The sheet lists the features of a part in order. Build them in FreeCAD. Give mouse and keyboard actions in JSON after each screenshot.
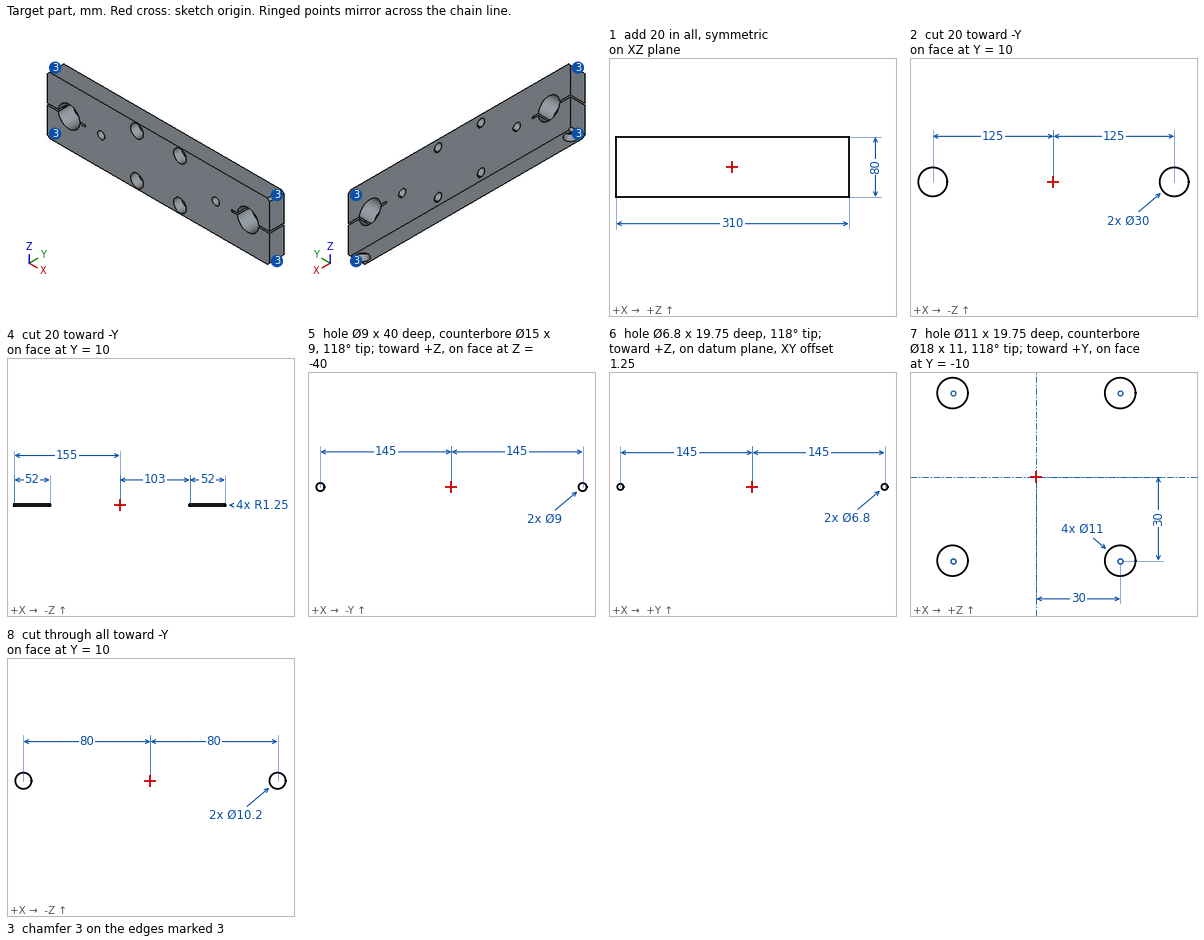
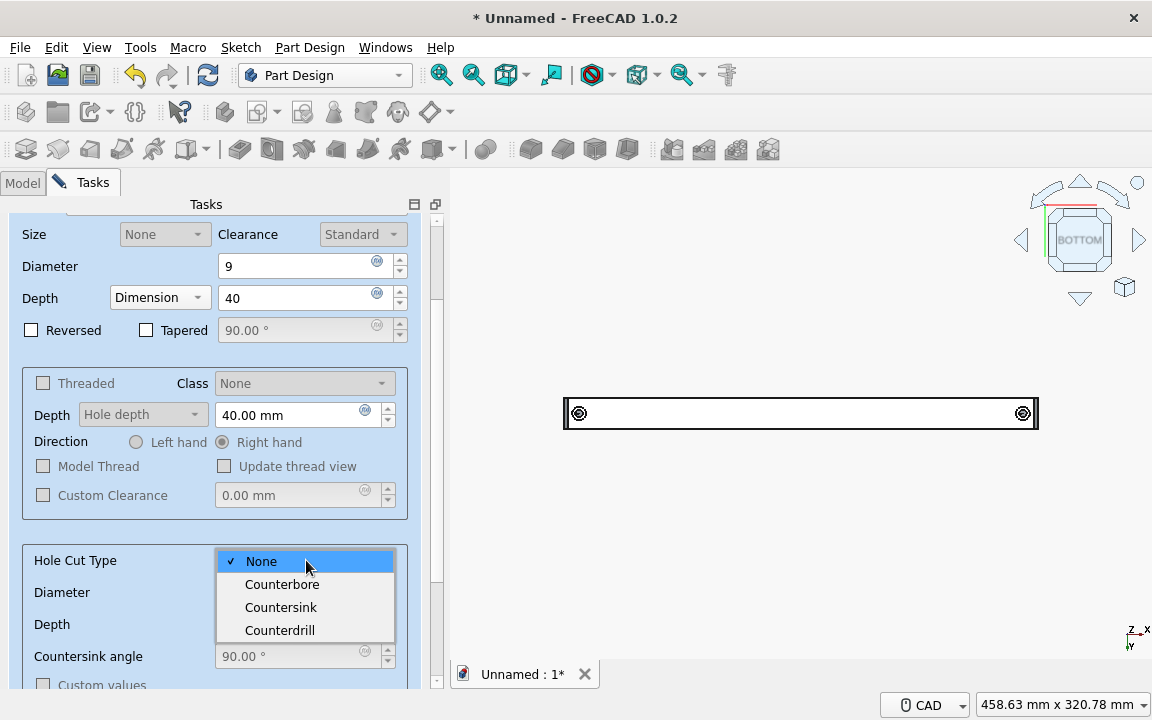
{"action": "left_click", "coordinate": [304, 584]}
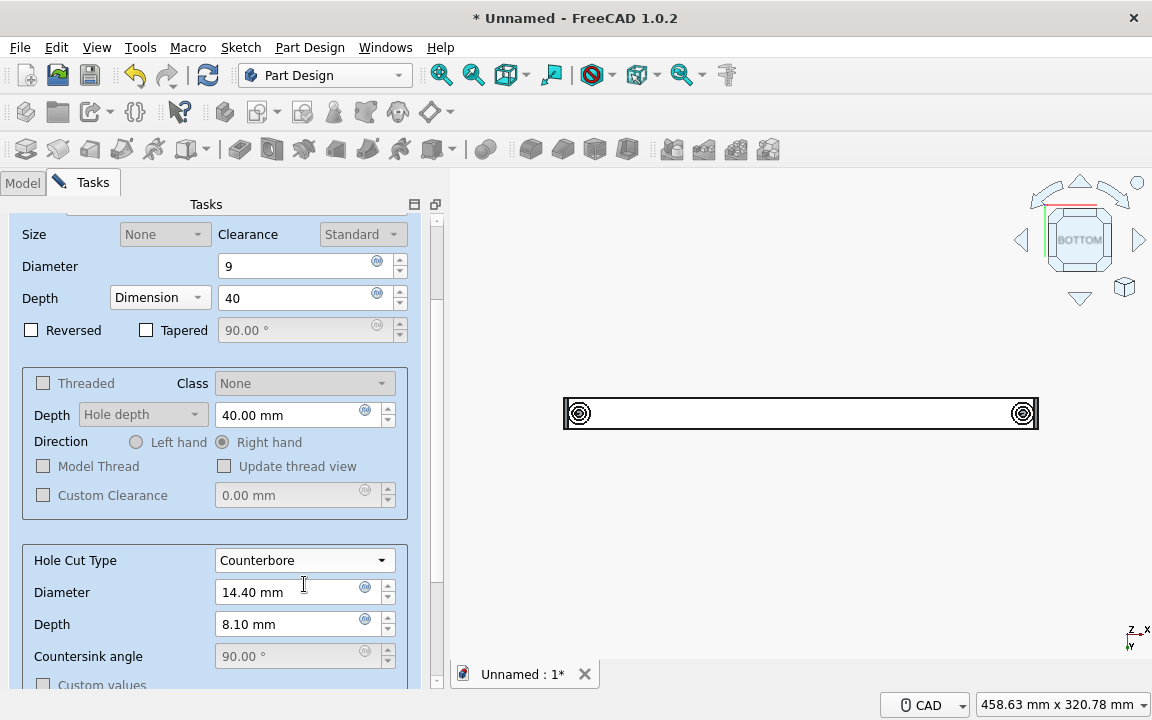
{"action": "triple_click", "coordinate": [298, 592]}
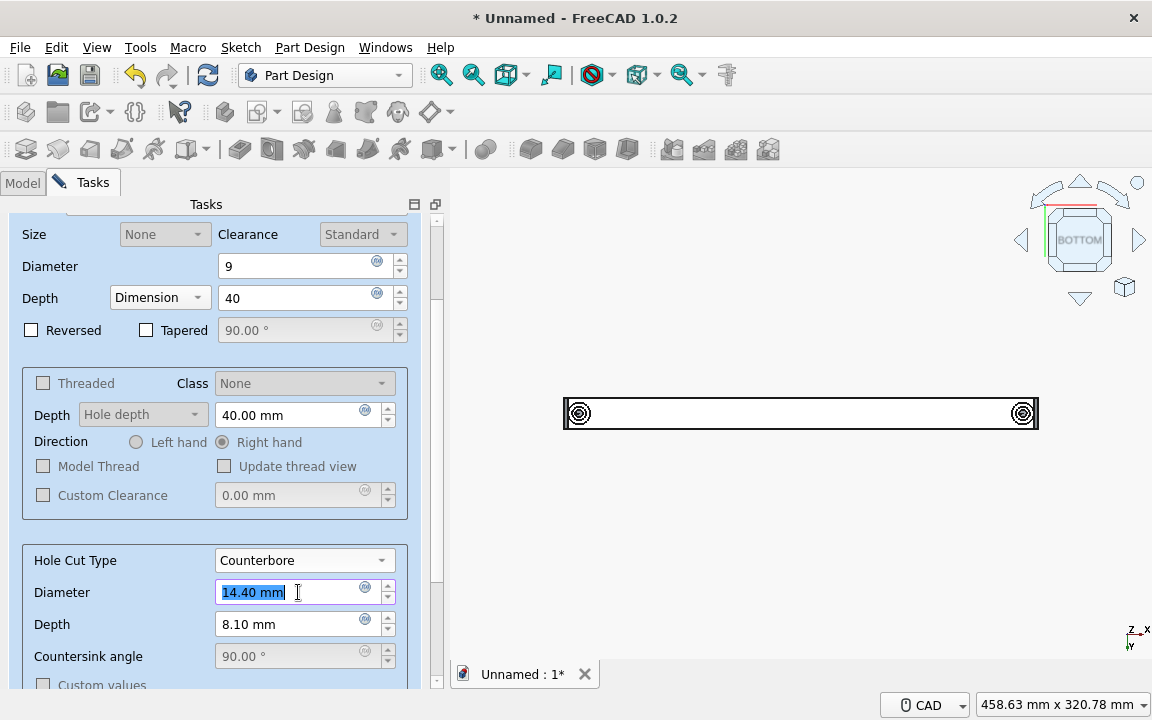
{"action": "type", "text": "15"}
{"action": "key", "text": "Tab"}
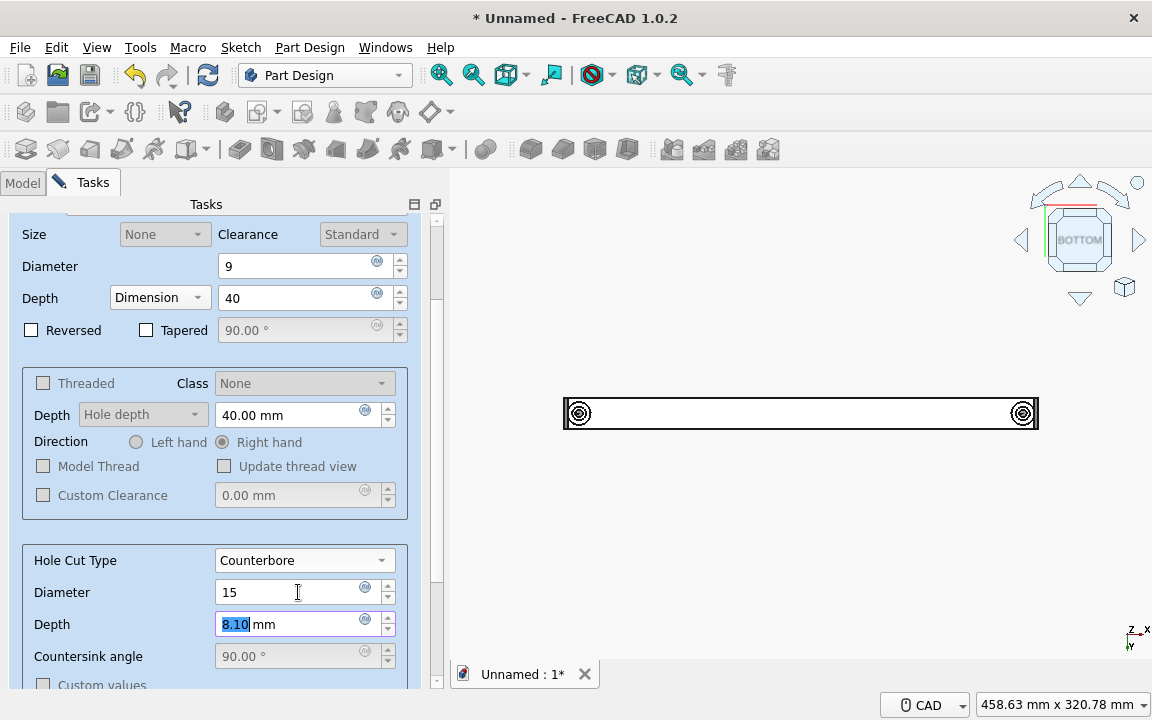
{"action": "type", "text": "9"}
{"action": "key", "text": "Tab"}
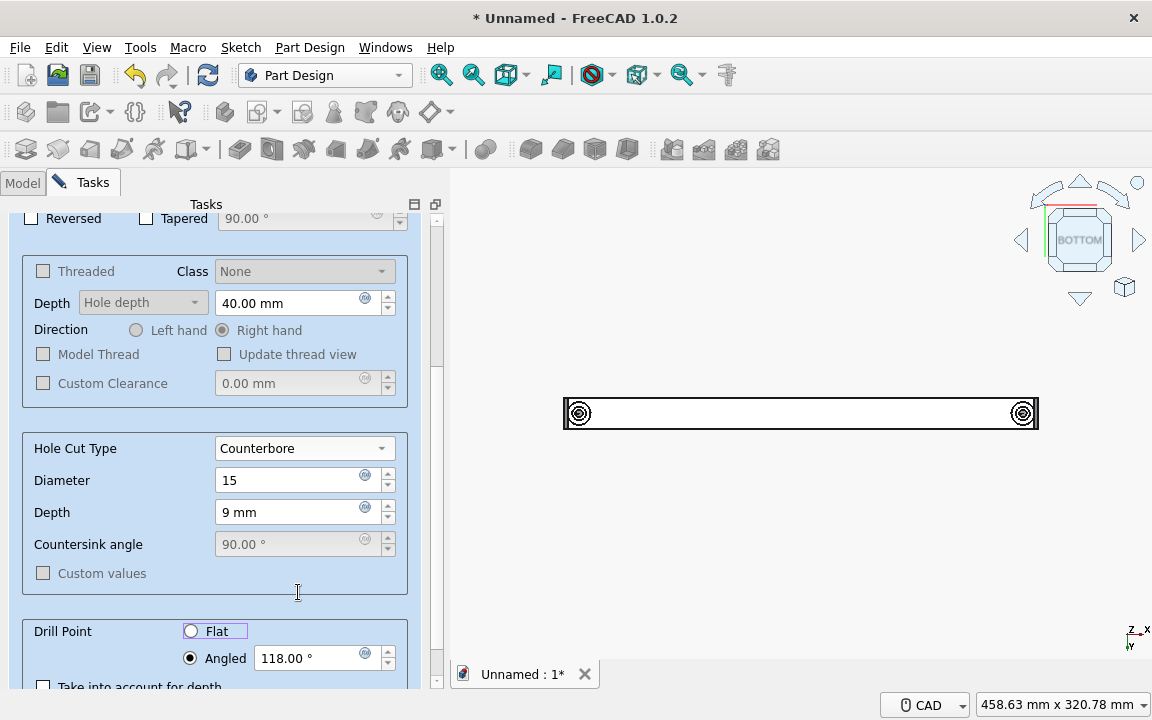
{"action": "scroll", "coordinate": [437, 451], "scroll_direction": "up", "scroll_amount": 5}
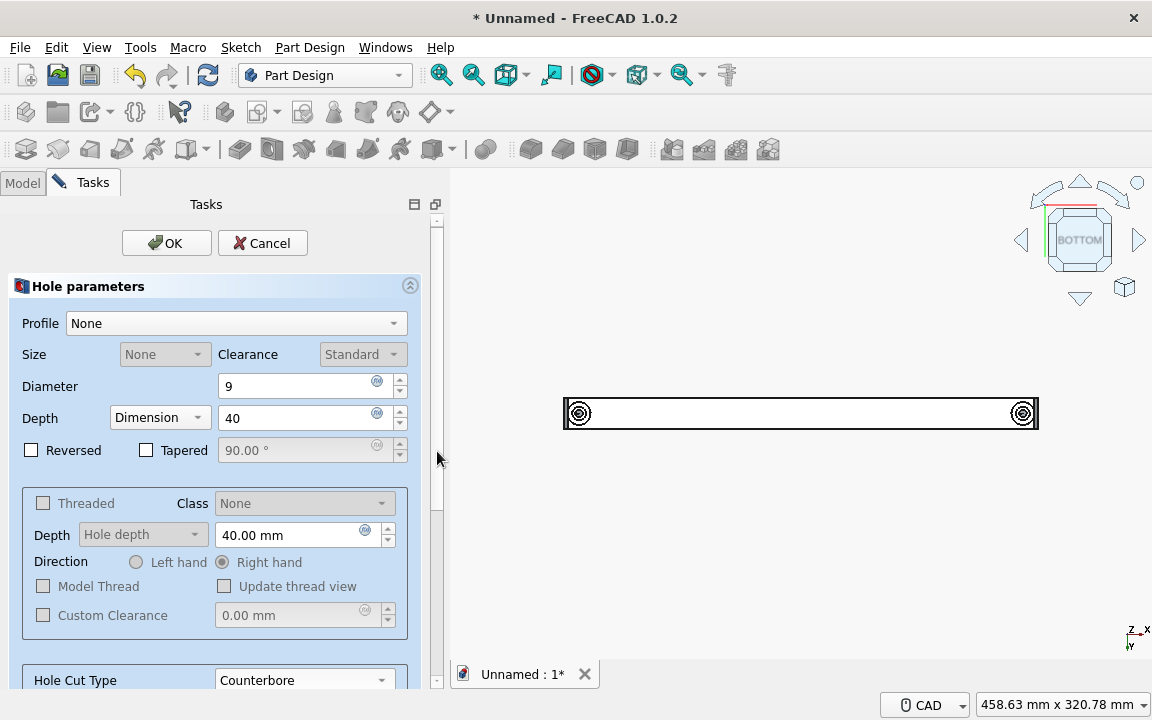
{"action": "left_click", "coordinate": [167, 243]}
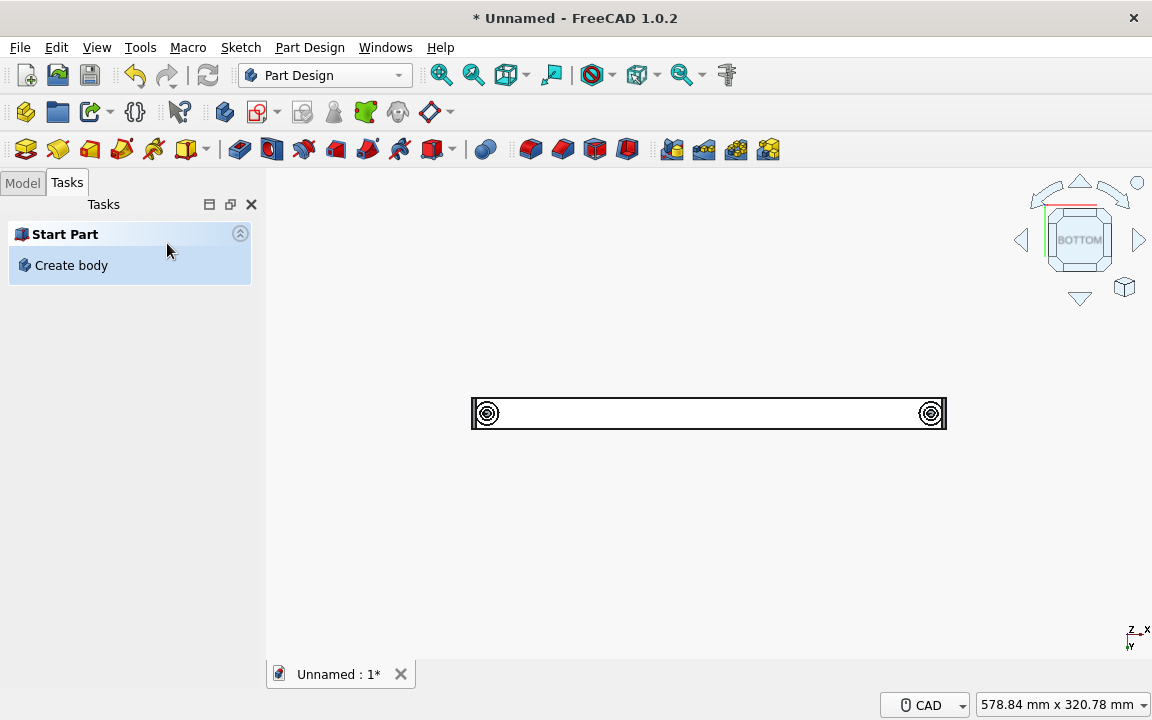
{"action": "left_click", "coordinate": [23, 182]}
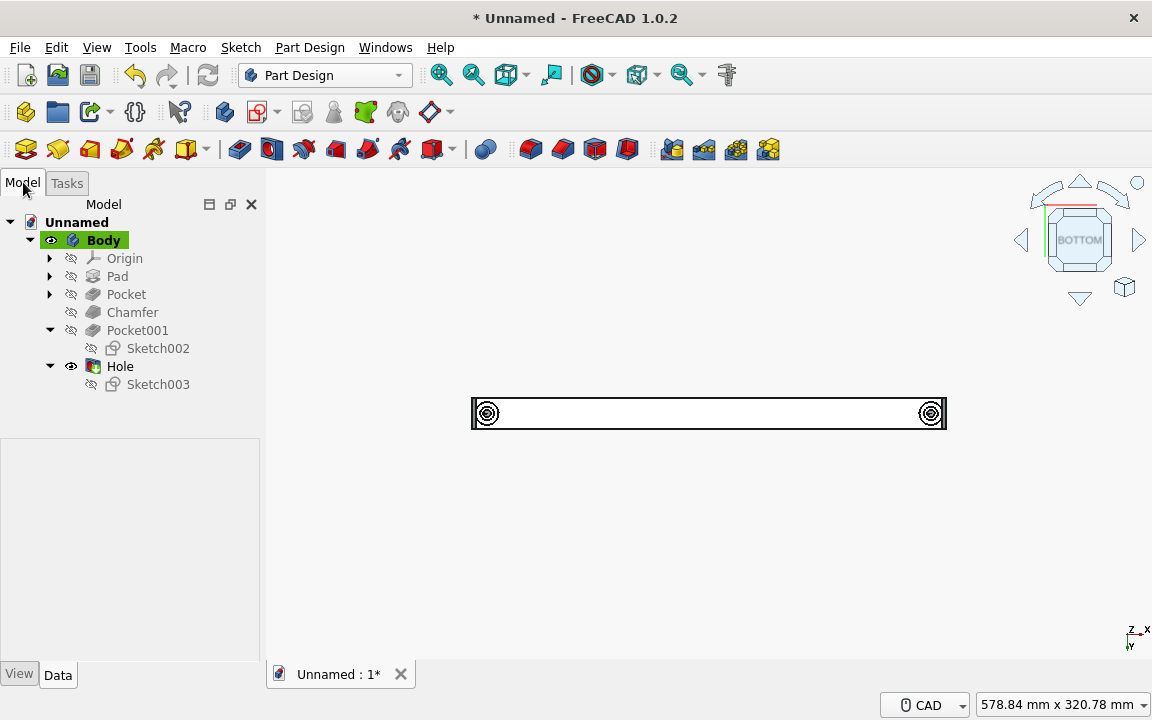
{"action": "left_click", "coordinate": [50, 258]}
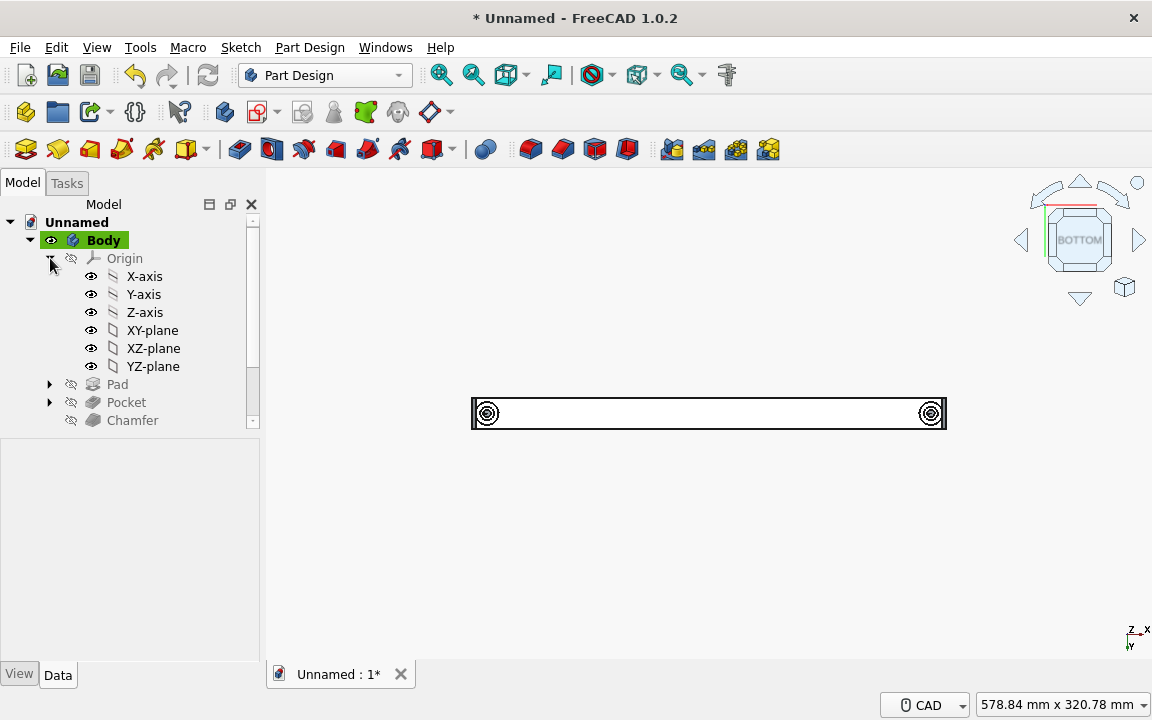
{"action": "left_click", "coordinate": [136, 330]}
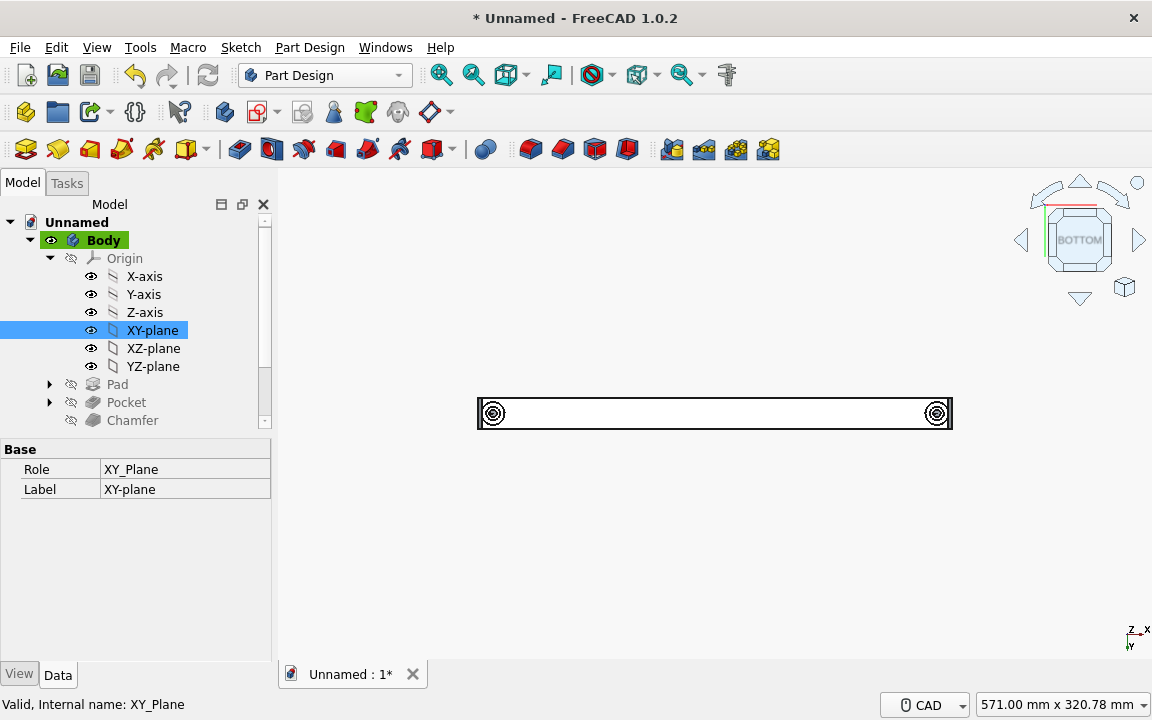
{"action": "left_click", "coordinate": [430, 112]}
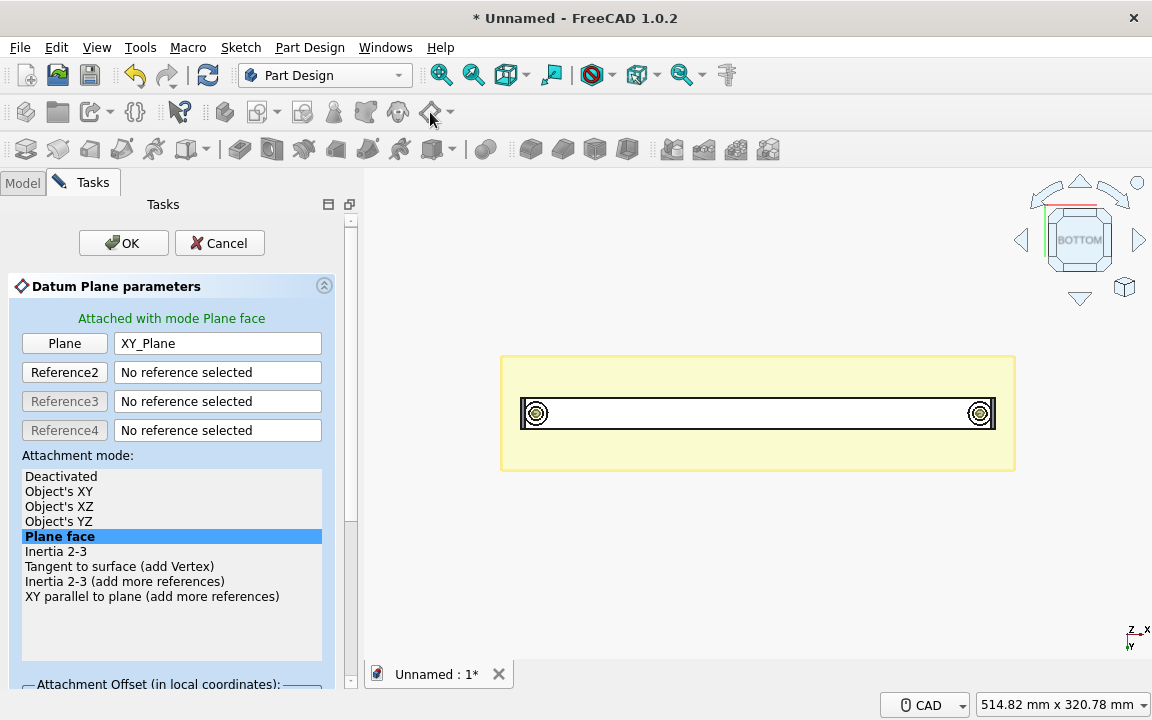
{"action": "scroll", "coordinate": [351, 451], "scroll_direction": "down", "scroll_amount": 3}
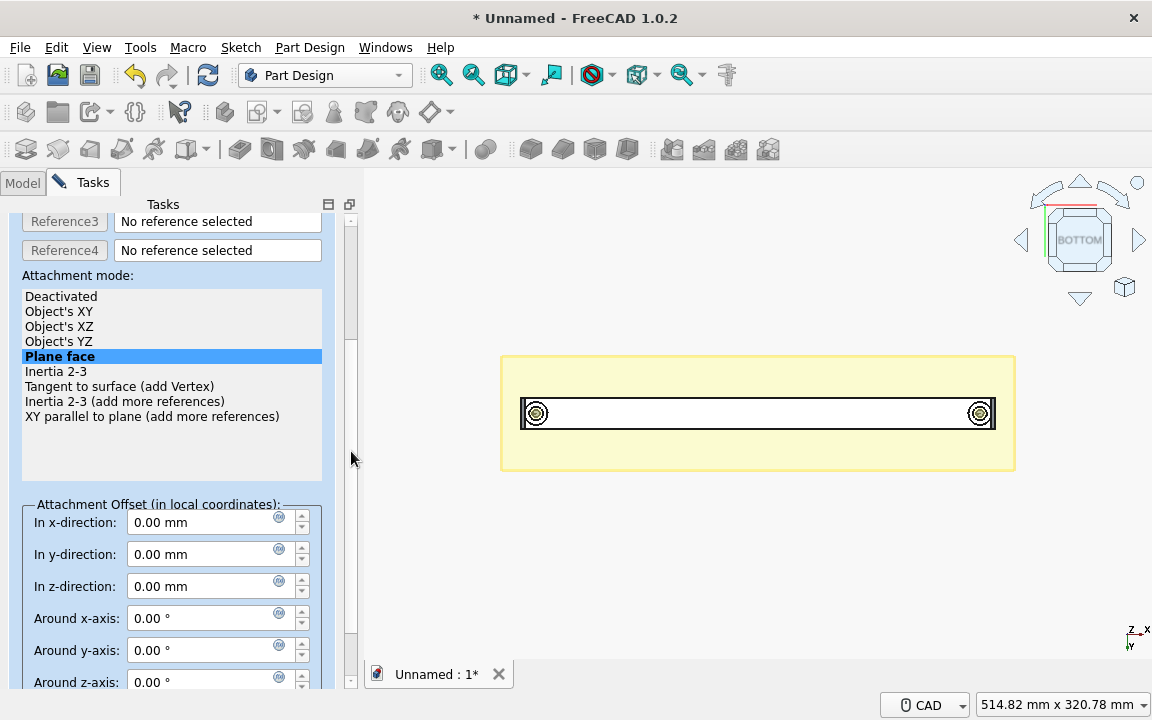
{"action": "triple_click", "coordinate": [210, 586]}